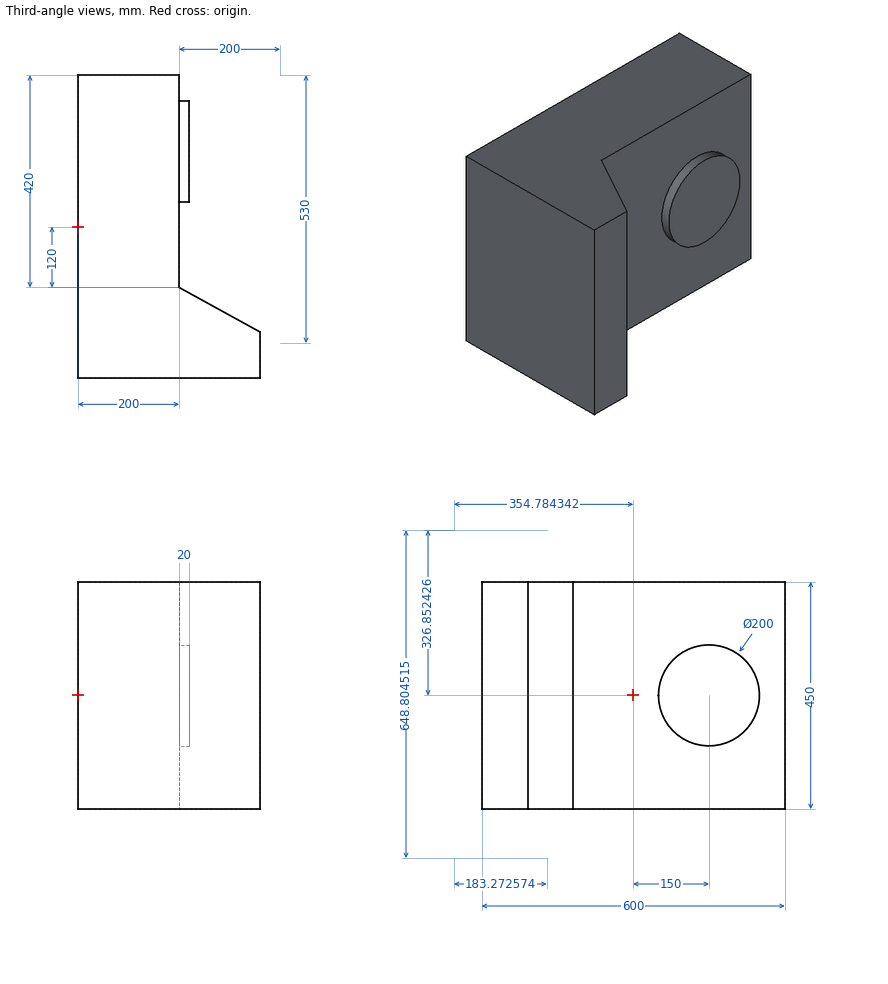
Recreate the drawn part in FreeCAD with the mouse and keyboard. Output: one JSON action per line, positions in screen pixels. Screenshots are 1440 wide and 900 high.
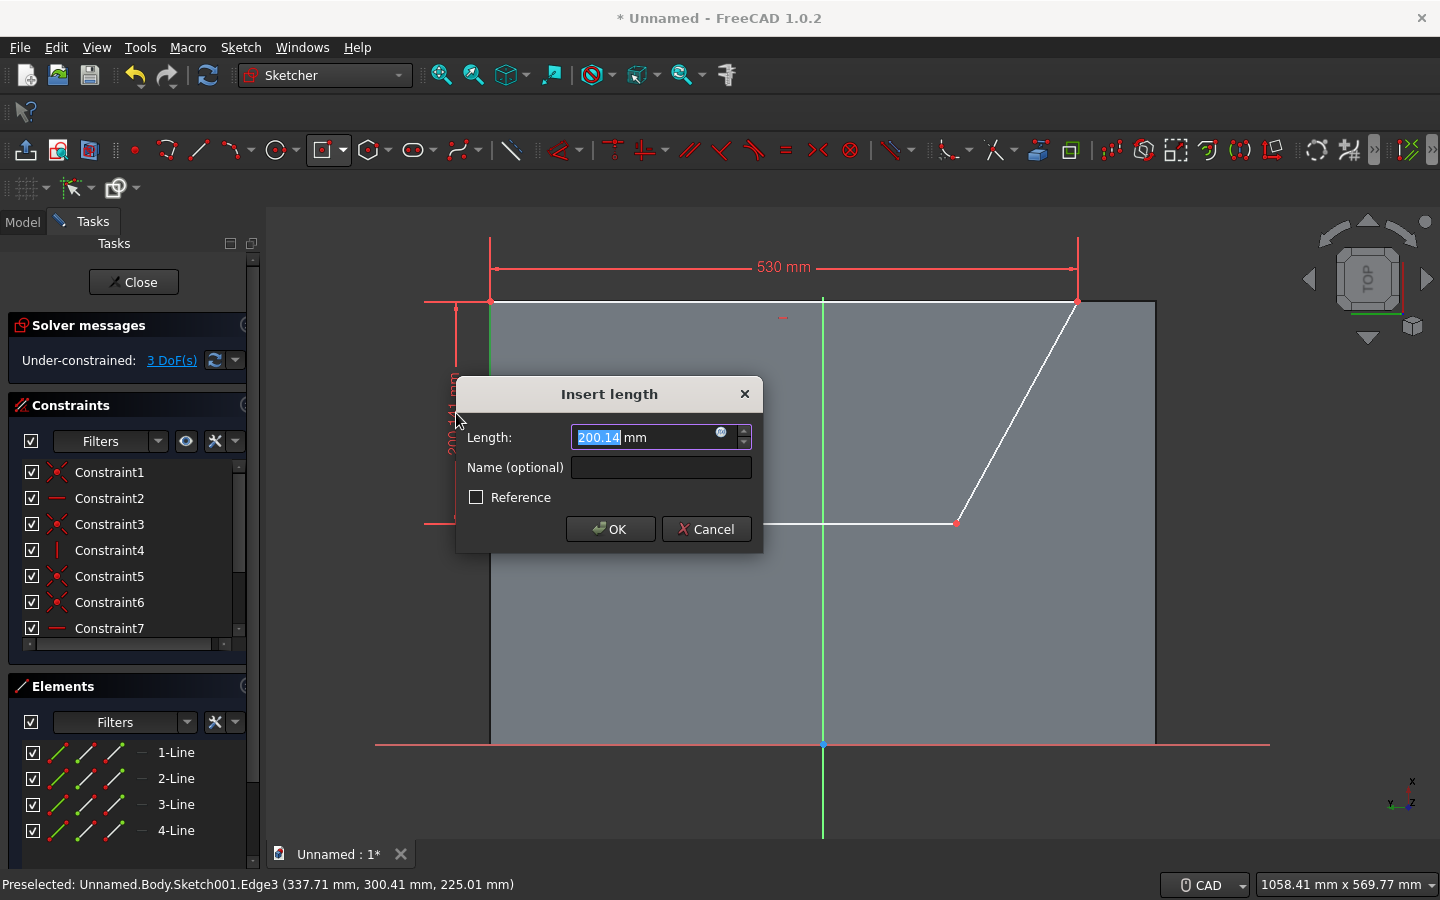
{"action": "type", "text": "200"}
{"action": "key", "text": "Return"}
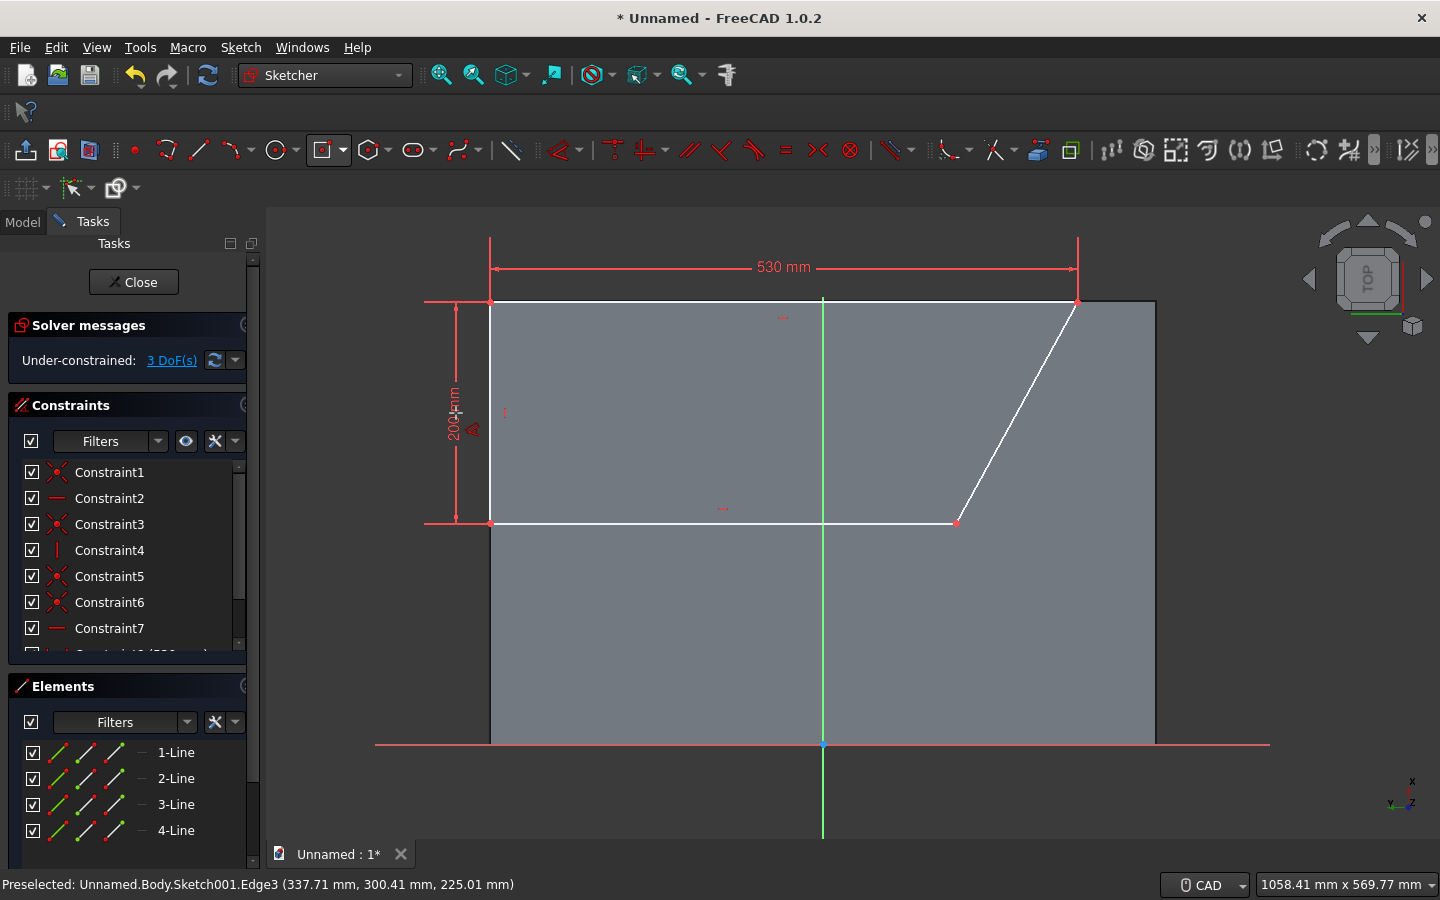
{"action": "left_click", "coordinate": [630, 524]}
{"action": "left_click", "coordinate": [723, 558]}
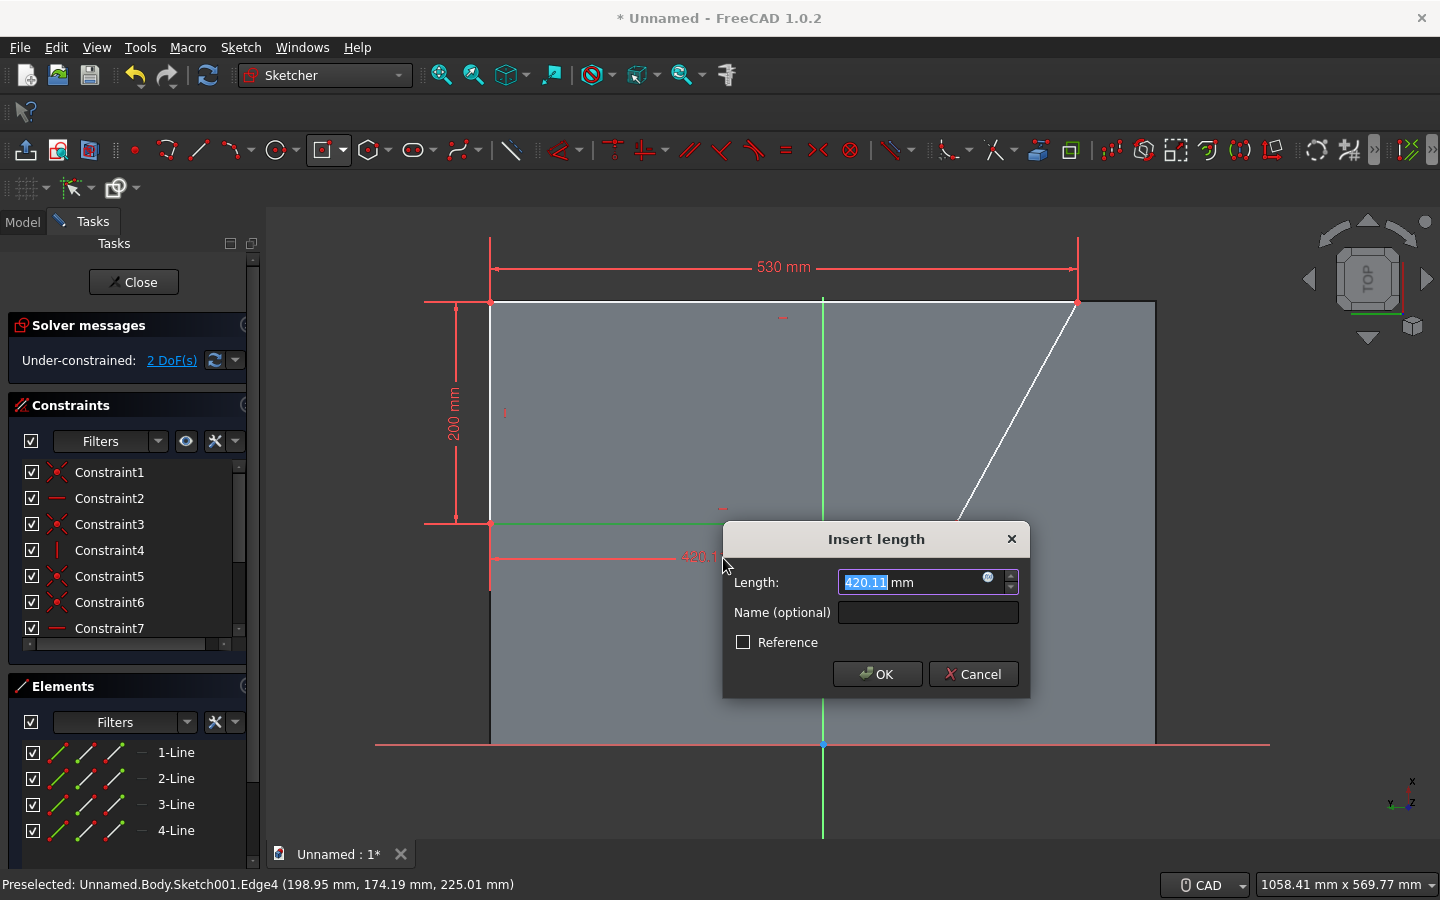
{"action": "type", "text": "420"}
{"action": "key", "text": "Return"}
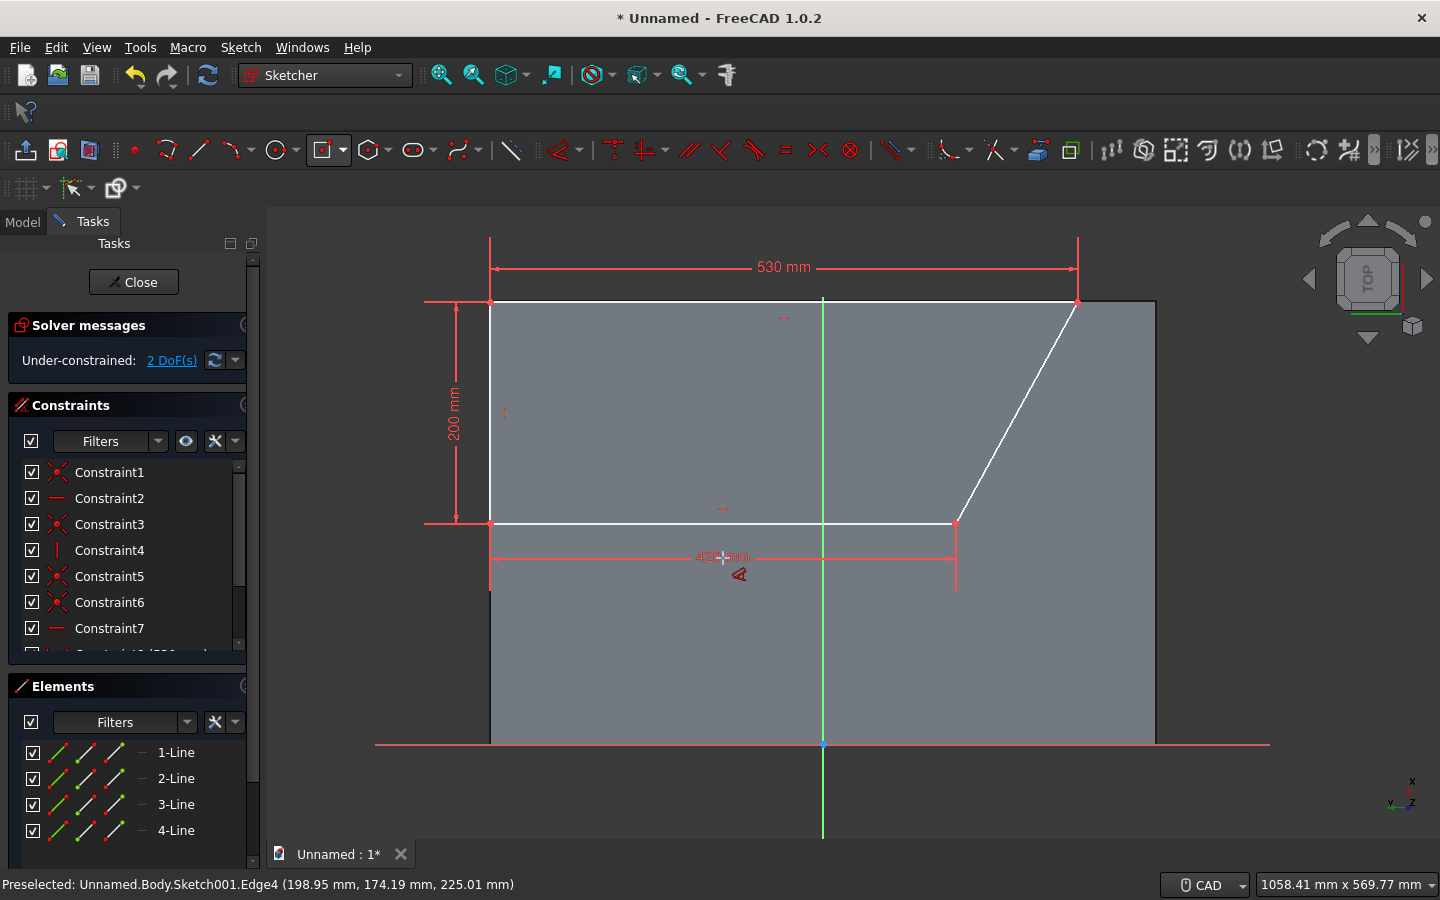
{"action": "left_click", "coordinate": [956, 524]}
{"action": "left_click", "coordinate": [890, 779]}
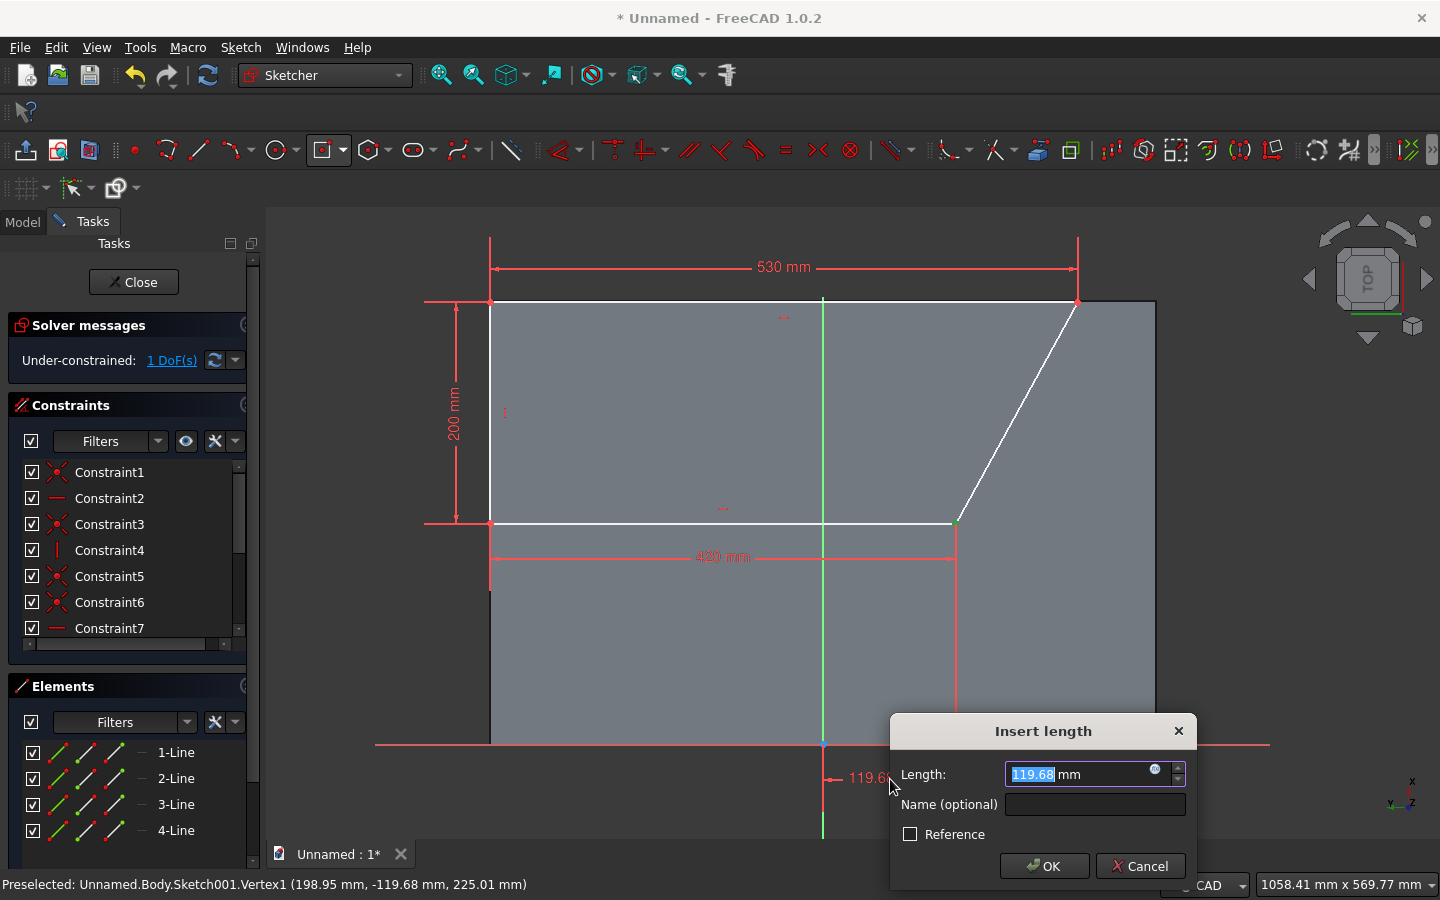
{"action": "type", "text": "120"}
{"action": "key", "text": "Return"}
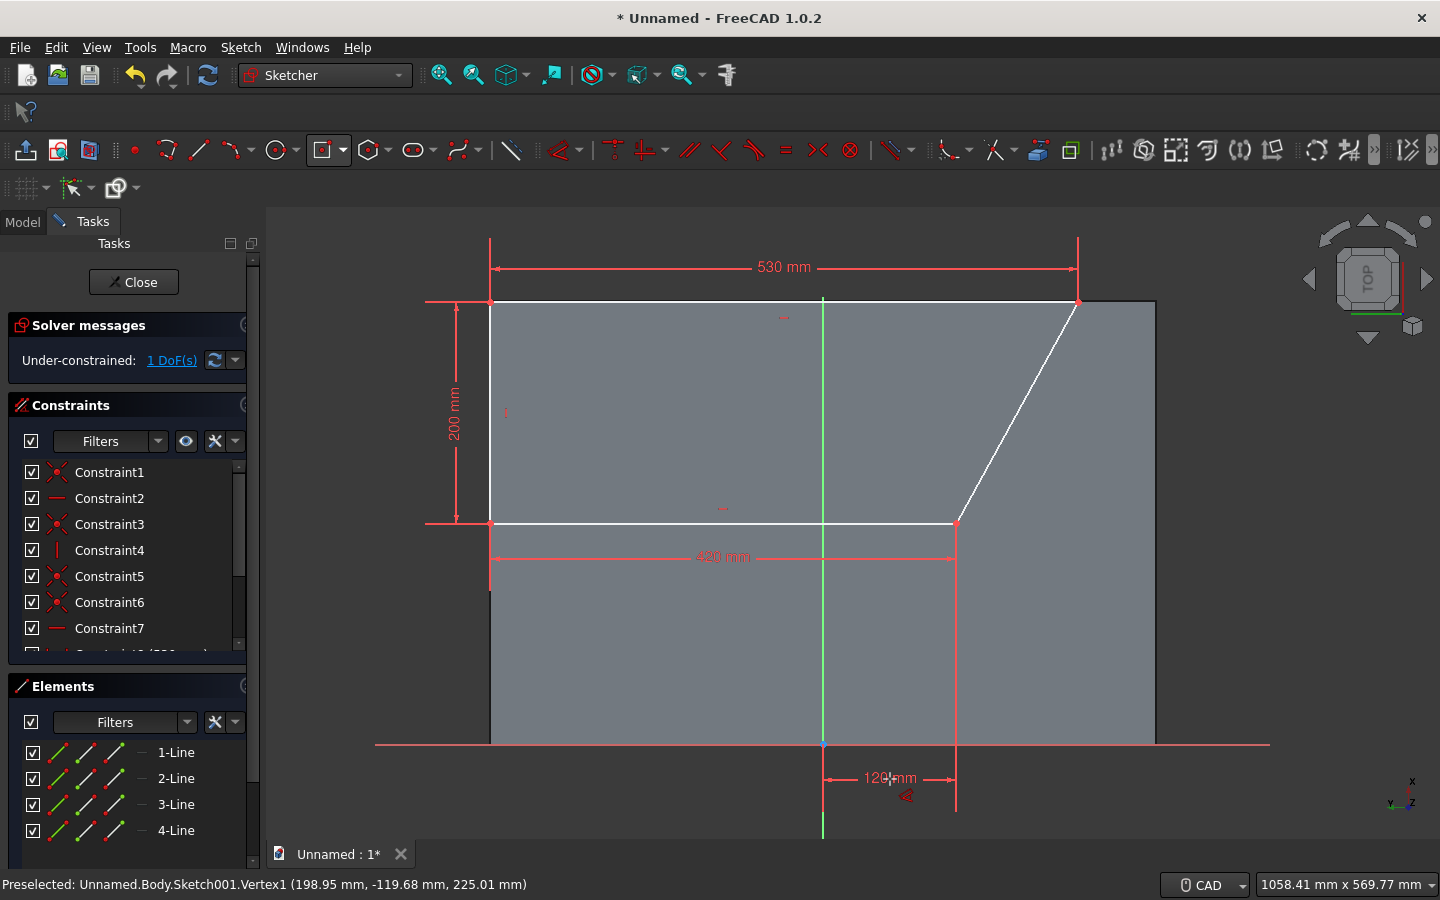
{"action": "left_click", "coordinate": [956, 524]}
{"action": "left_click", "coordinate": [990, 634]}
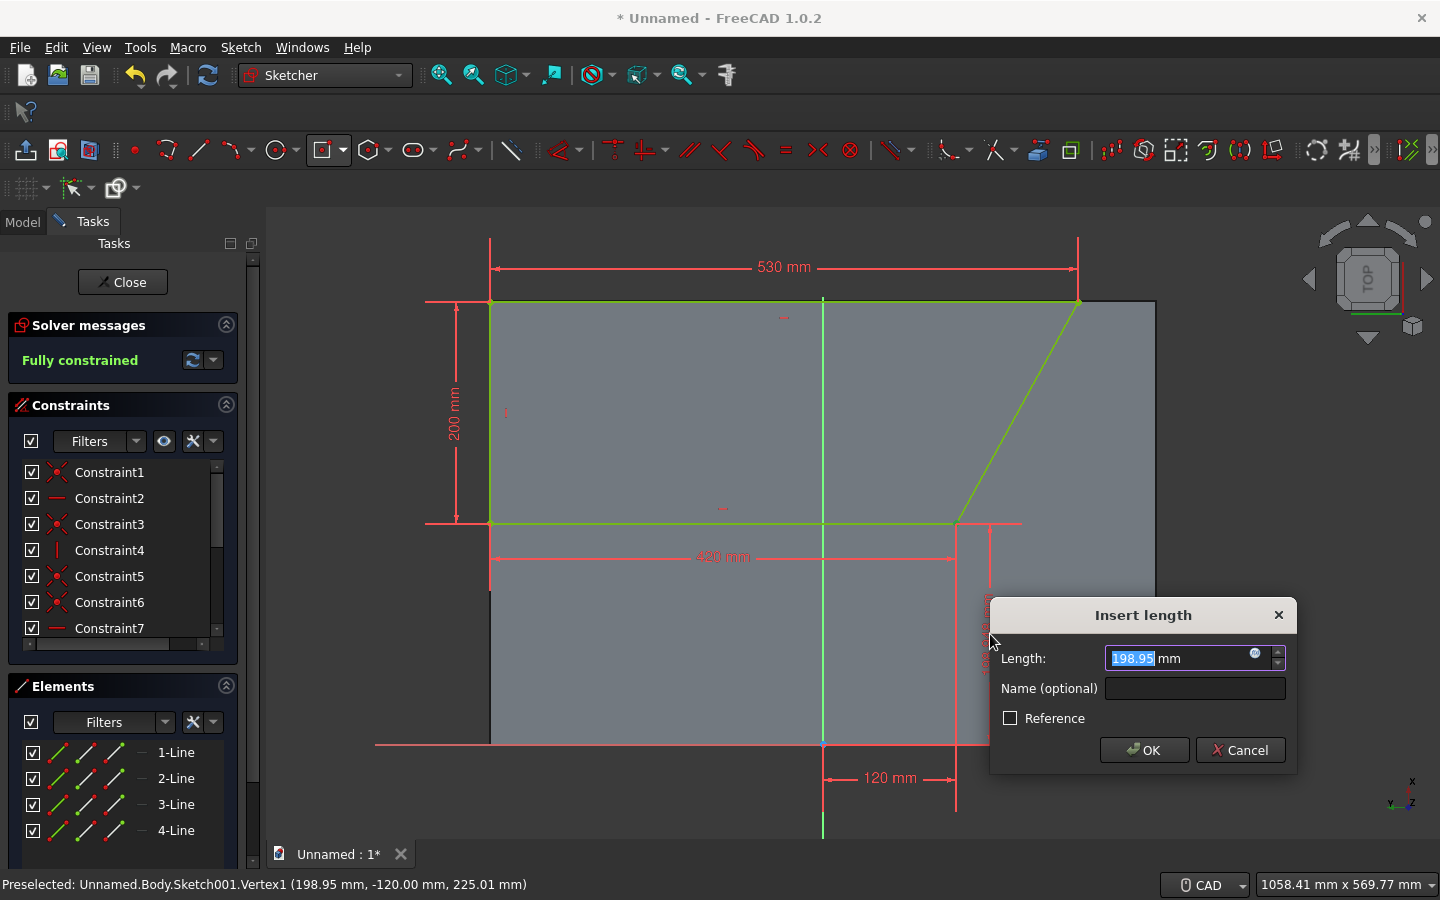
{"action": "type", "text": "200"}
{"action": "key", "text": "Return"}
{"action": "key", "text": "Escape"}